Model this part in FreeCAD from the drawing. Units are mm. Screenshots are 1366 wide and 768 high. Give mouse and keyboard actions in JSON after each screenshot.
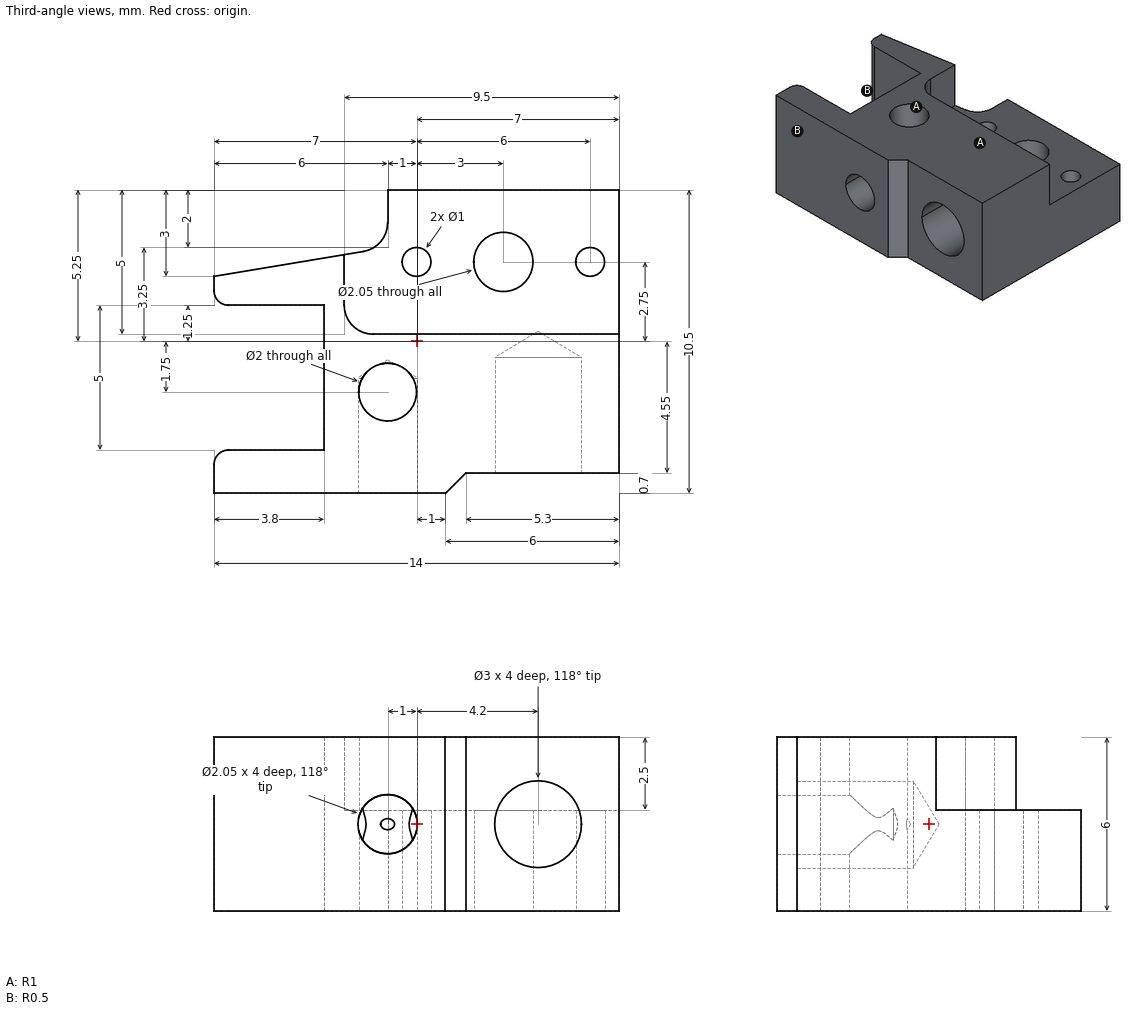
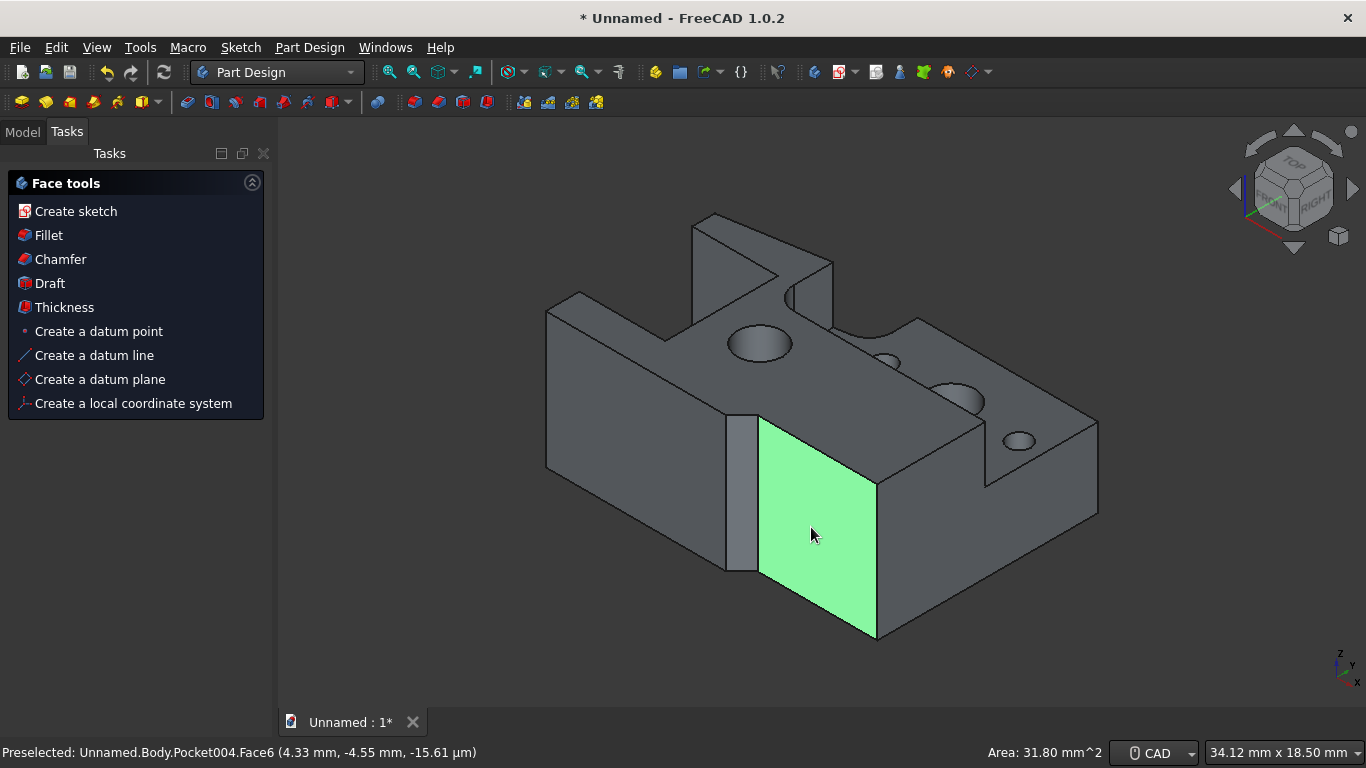
{"action": "left_click", "coordinate": [840, 72]}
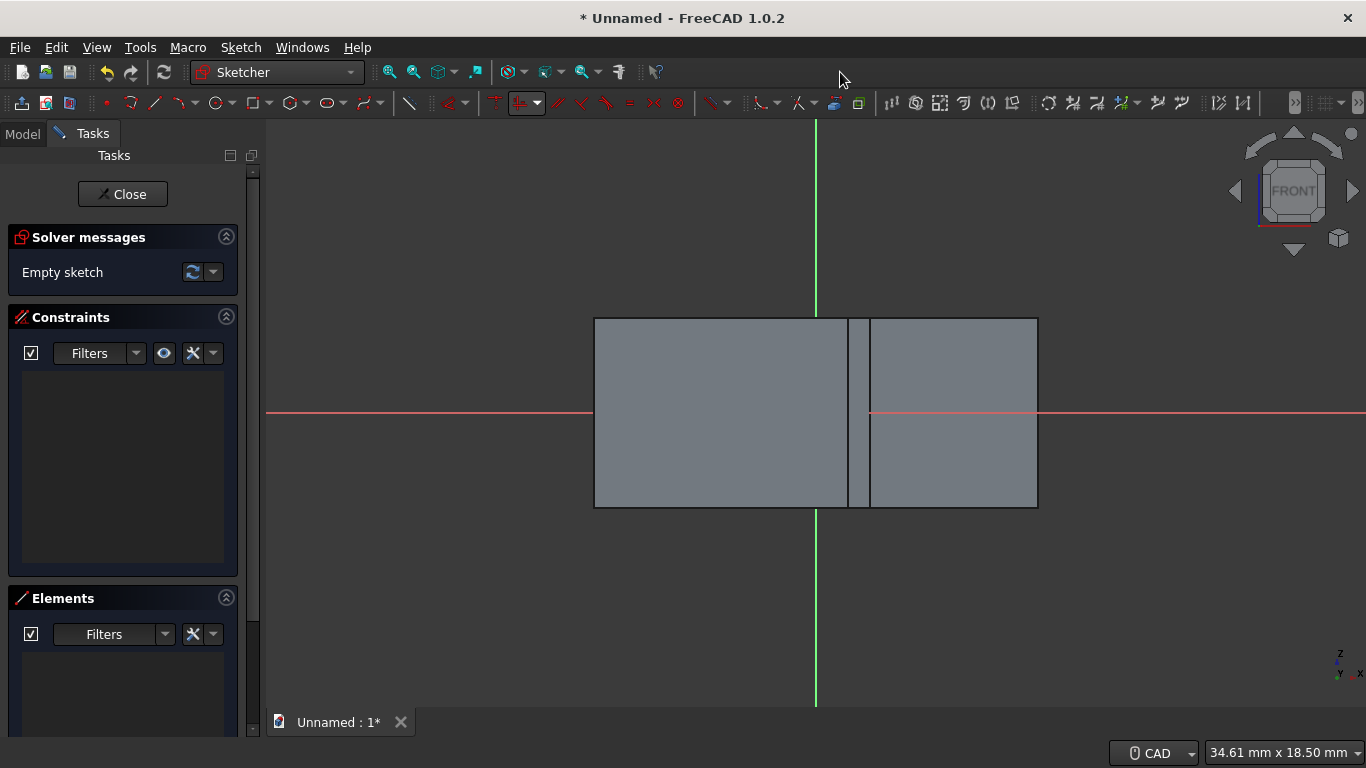
{"action": "scroll", "coordinate": [975, 413], "scroll_direction": "up", "scroll_amount": 6}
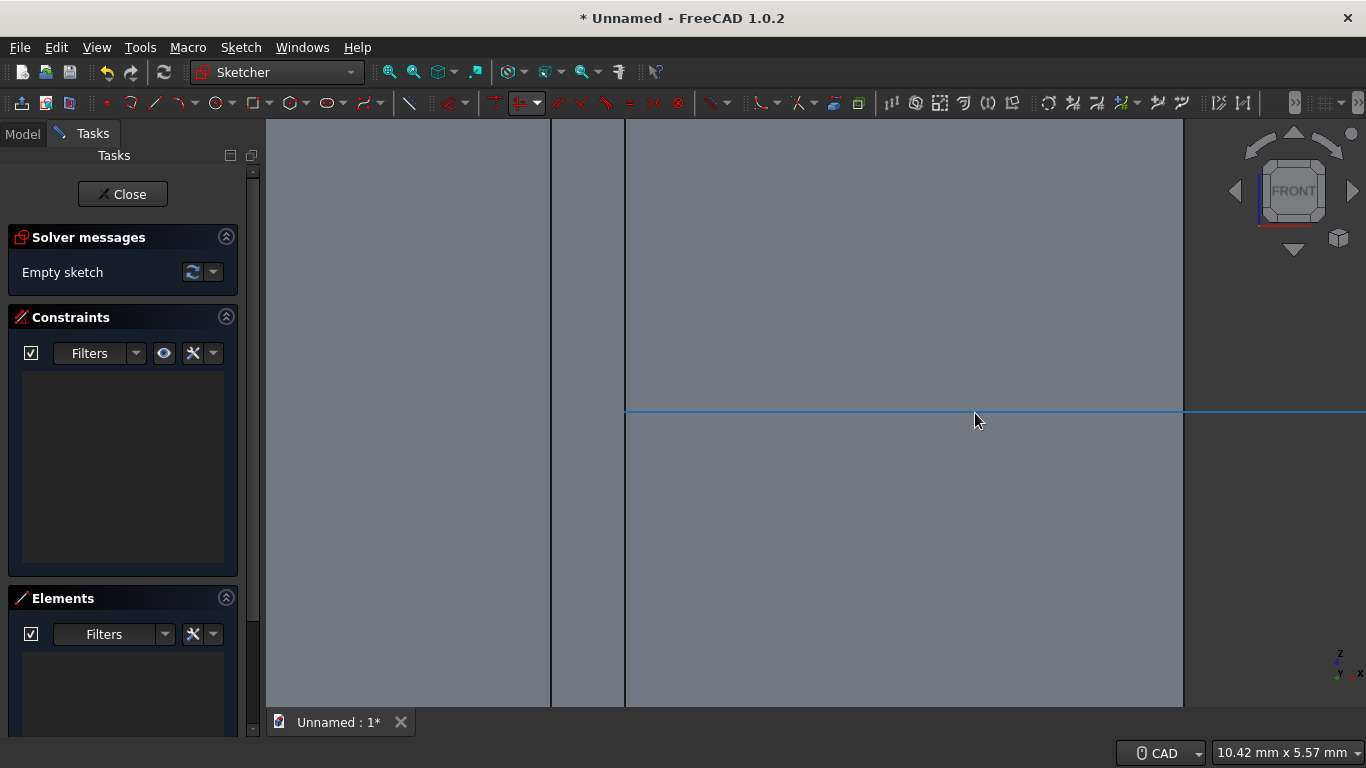
{"action": "left_click", "coordinate": [216, 104]}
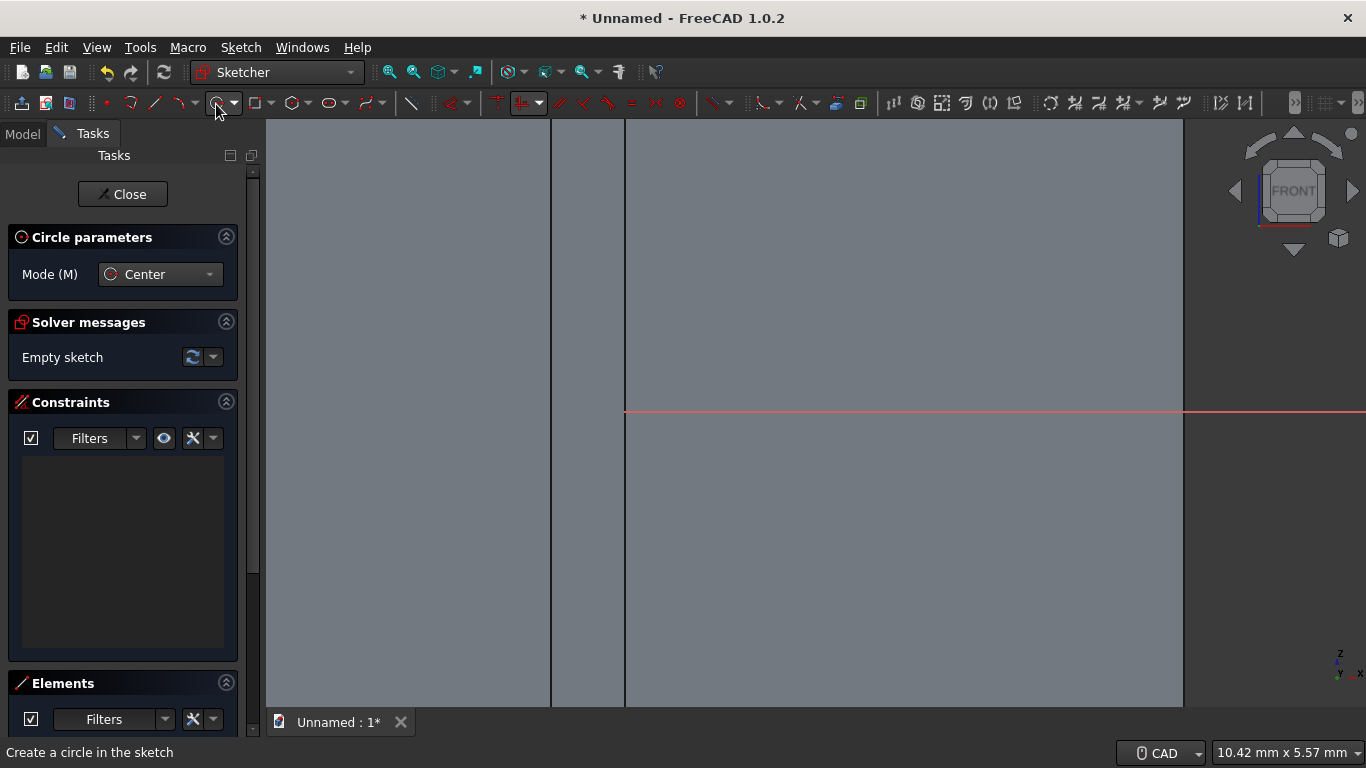
{"action": "left_click", "coordinate": [889, 412]}
{"action": "left_click", "coordinate": [1001, 300]}
{"action": "key", "text": "Escape"}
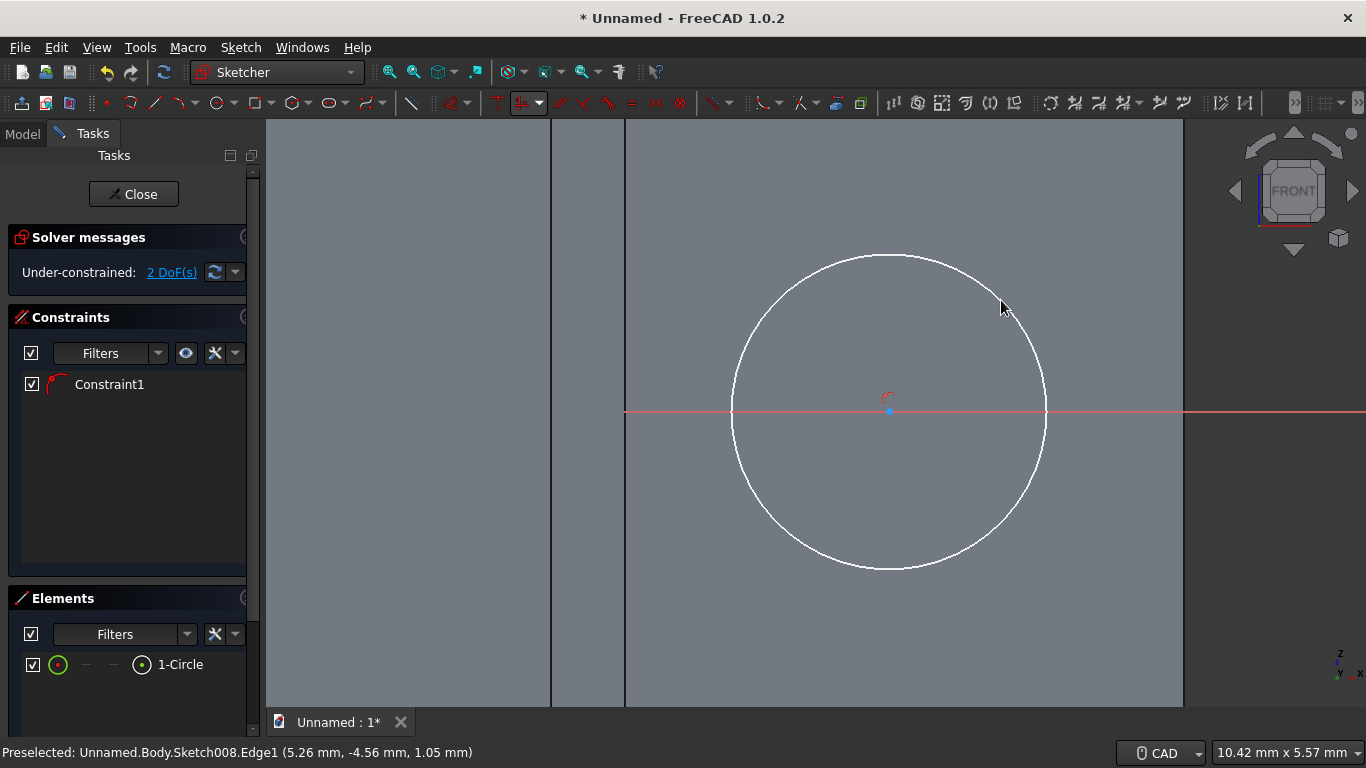
{"action": "left_click", "coordinate": [450, 104]}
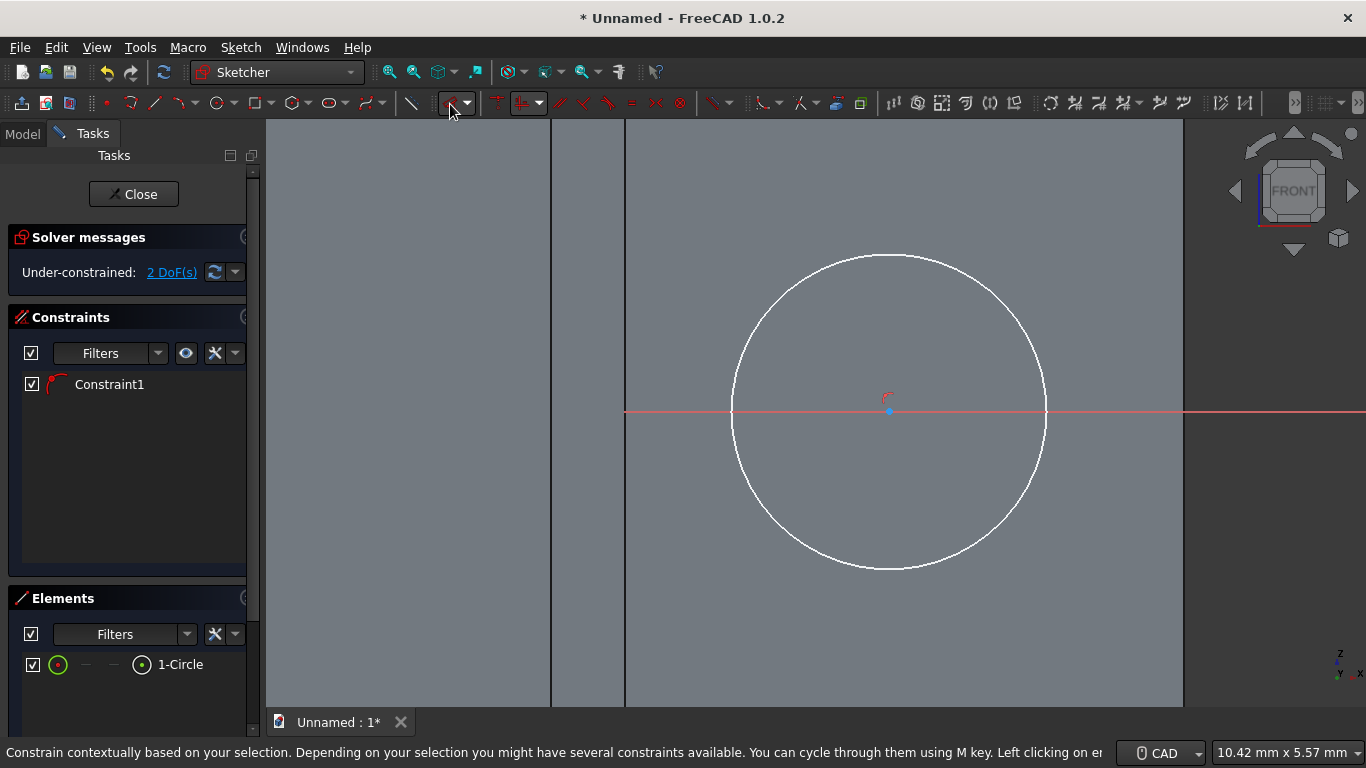
{"action": "left_click", "coordinate": [1000, 300]}
{"action": "left_click", "coordinate": [1023, 277]}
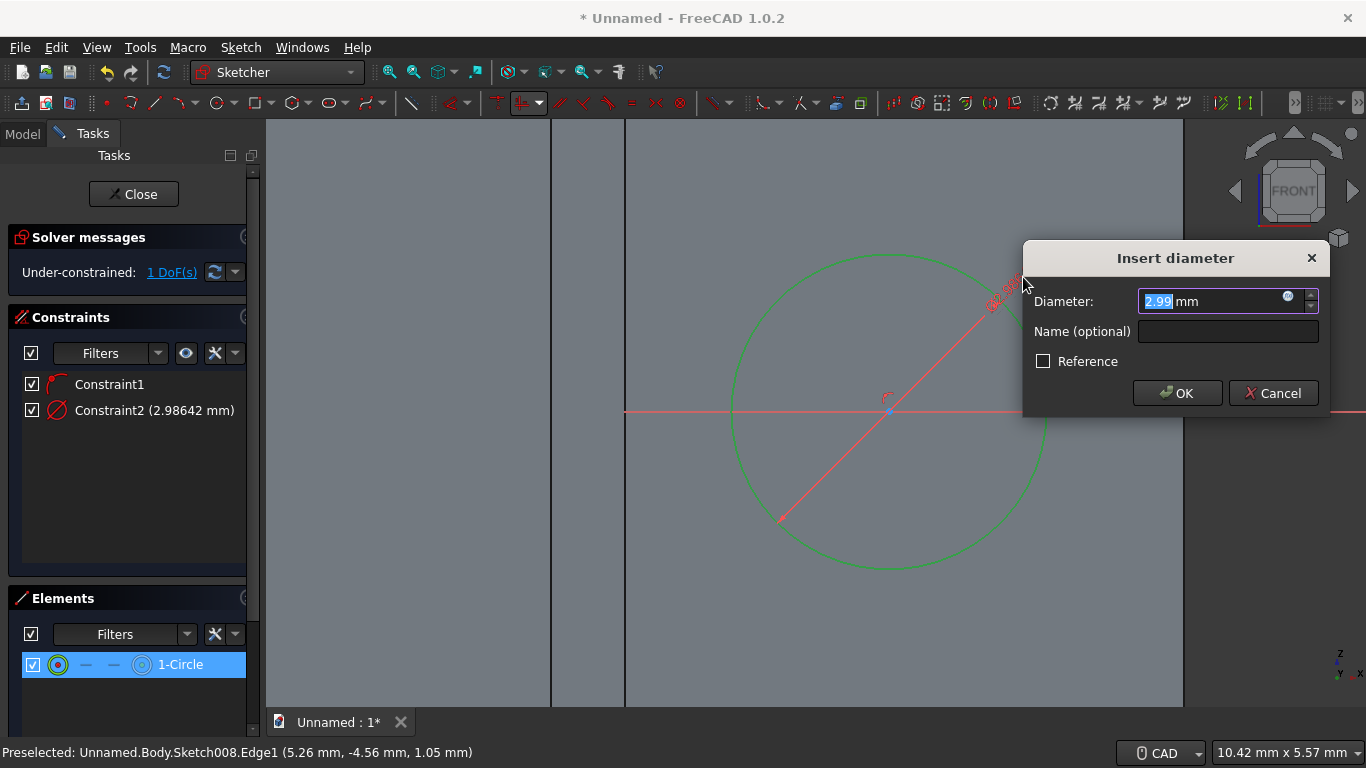
{"action": "type", "text": "3"}
{"action": "key", "text": "Return"}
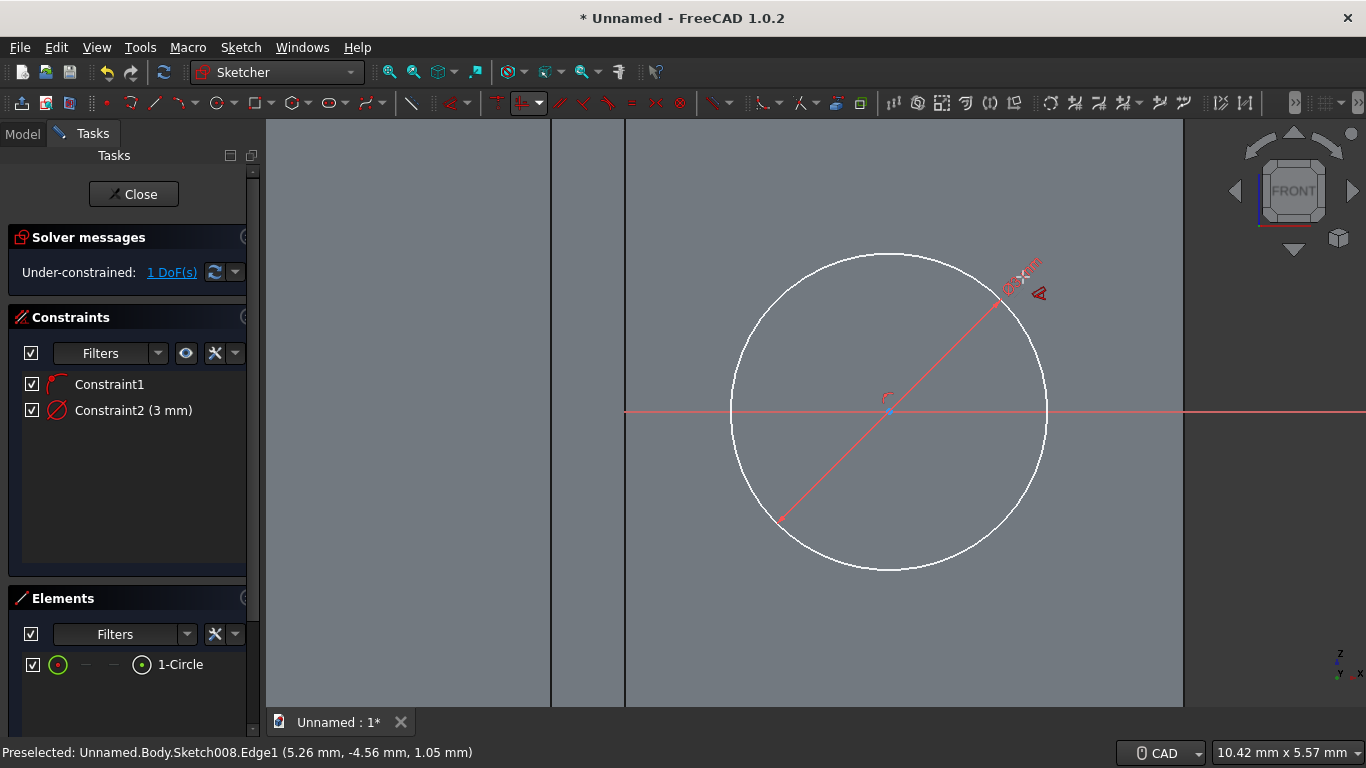
{"action": "left_click", "coordinate": [889, 412]}
{"action": "left_click", "coordinate": [667, 446]}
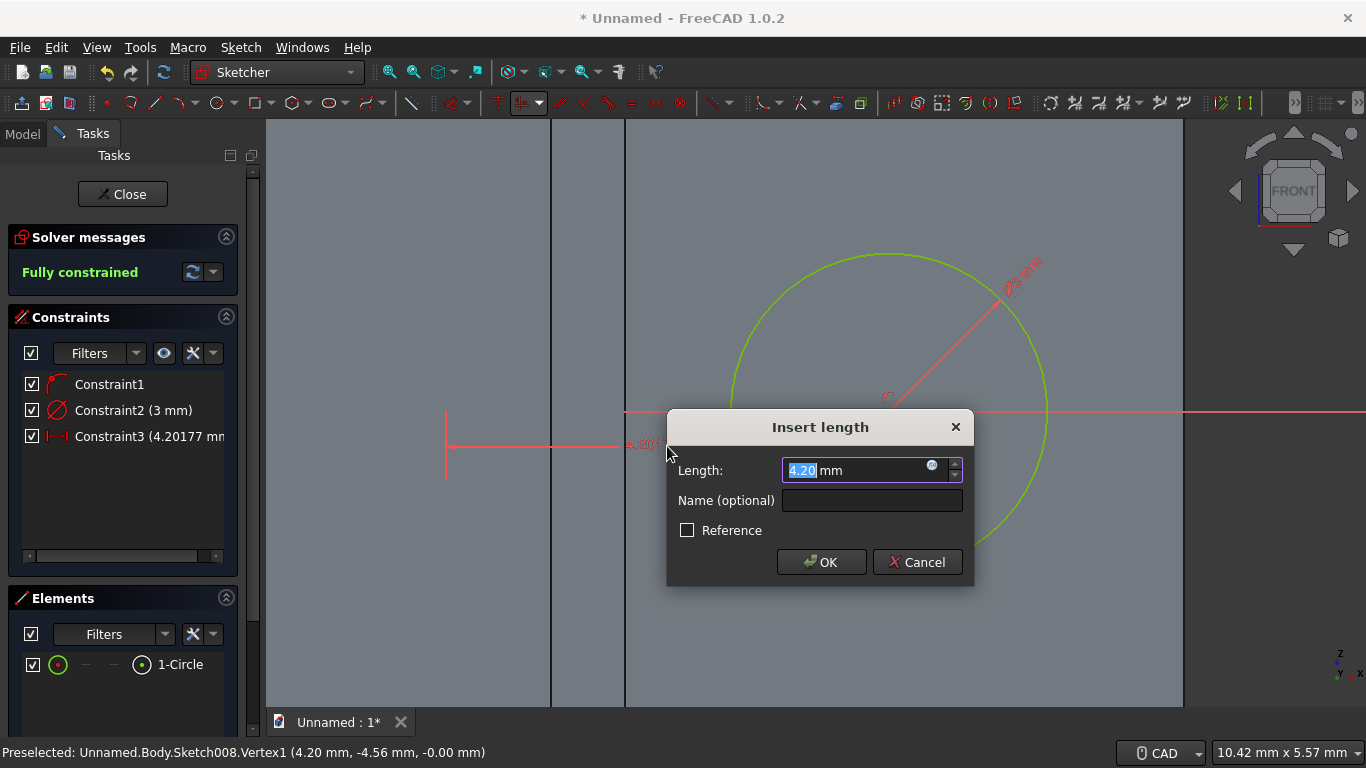
{"action": "type", "text": "4.2"}
{"action": "key", "text": "Return"}
{"action": "key", "text": "Escape"}